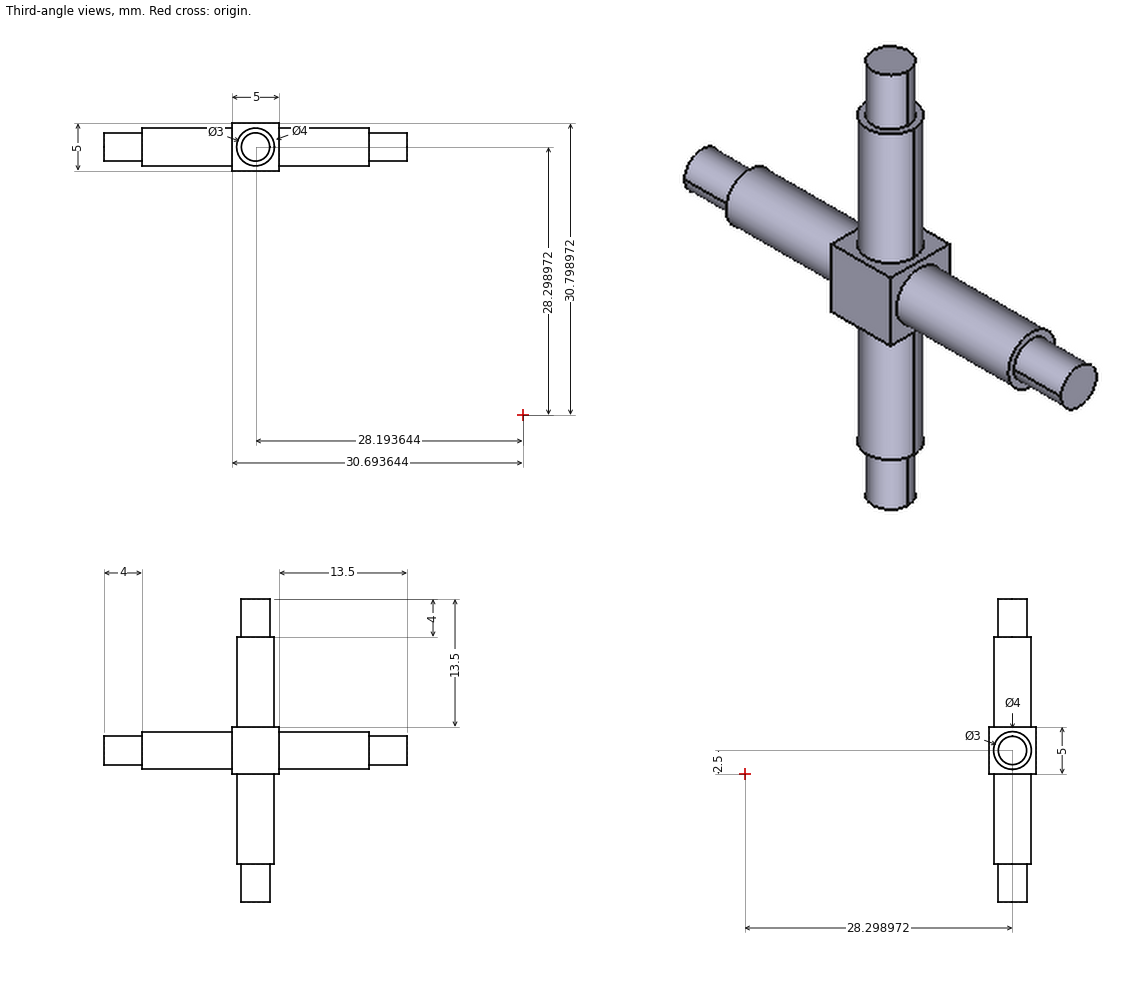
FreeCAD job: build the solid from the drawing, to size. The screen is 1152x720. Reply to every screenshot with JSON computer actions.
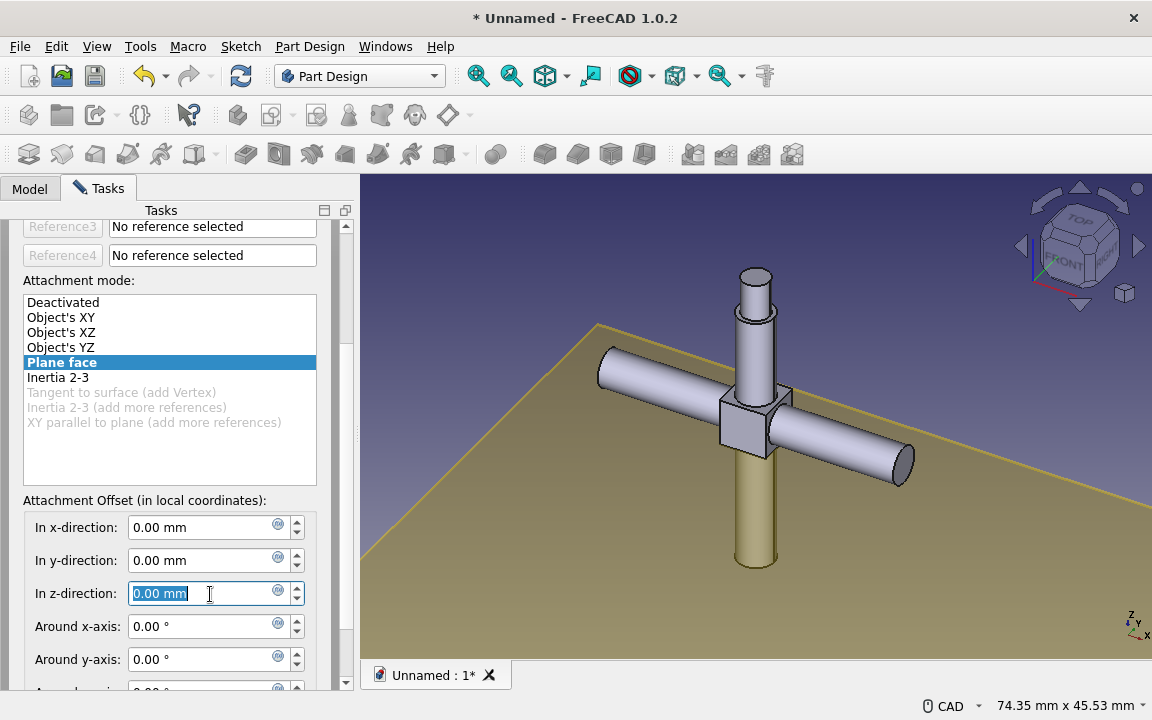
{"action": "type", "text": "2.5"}
{"action": "key", "text": "Tab"}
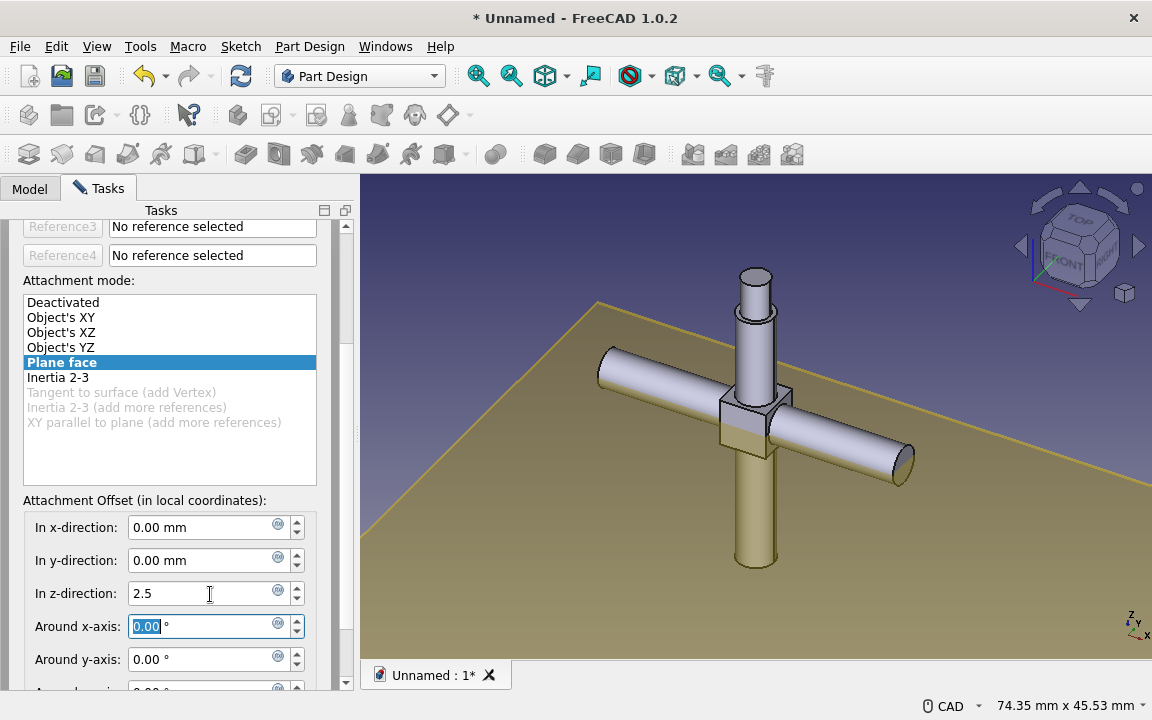
{"action": "scroll", "coordinate": [346, 455], "scroll_direction": "up", "scroll_amount": 4}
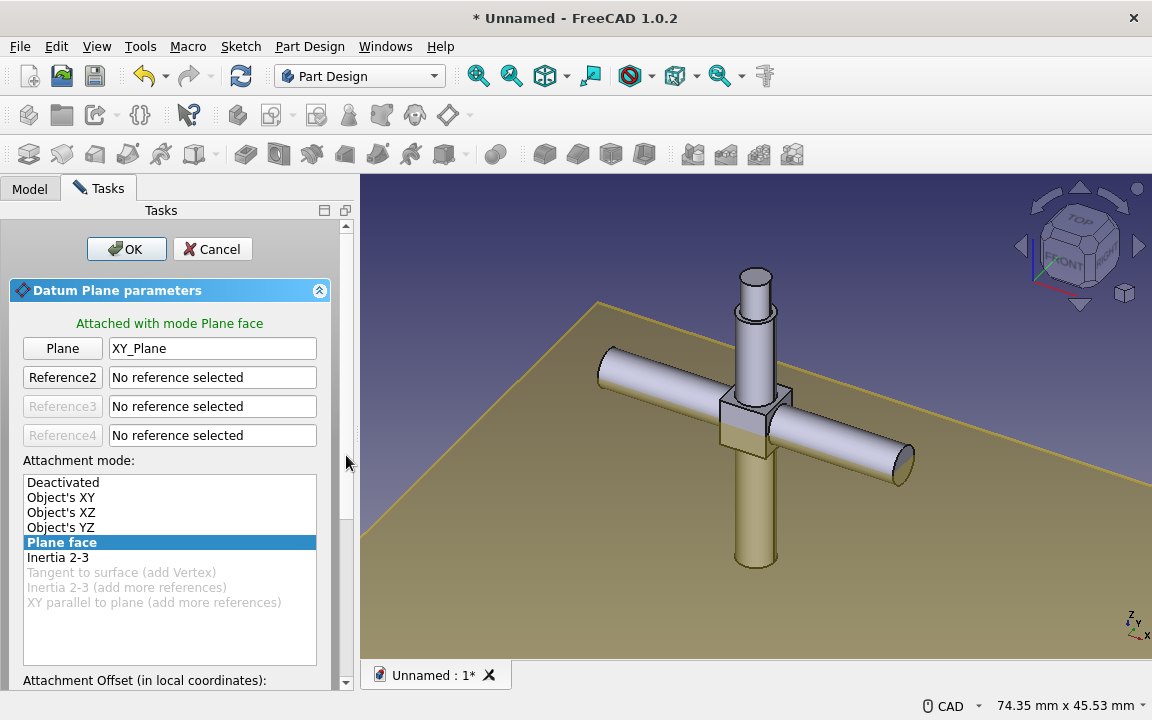
{"action": "left_click", "coordinate": [127, 249]}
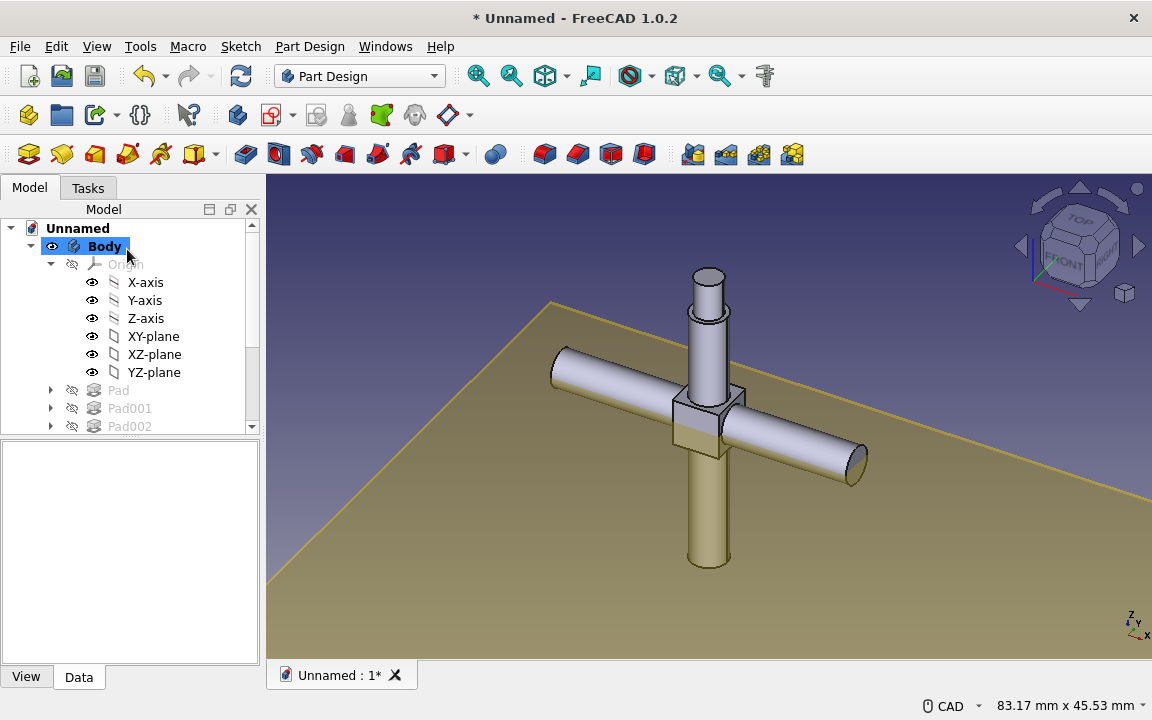
{"action": "scroll", "coordinate": [101, 332], "scroll_direction": "down", "scroll_amount": 3}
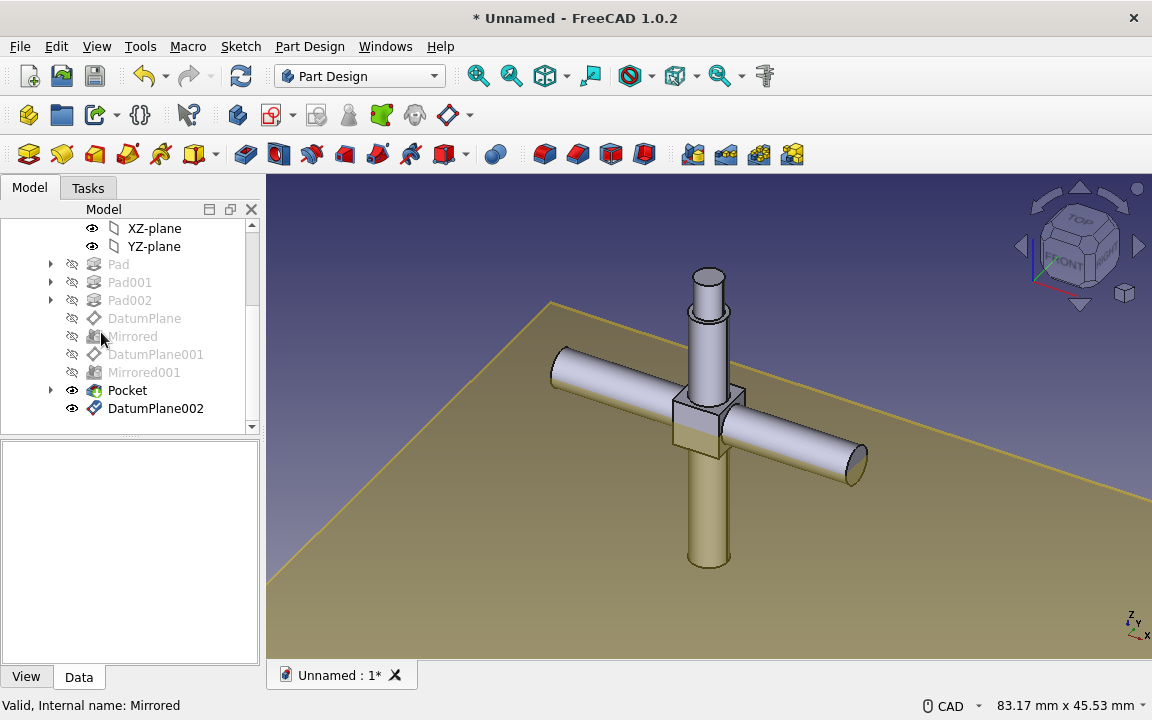
{"action": "left_click", "coordinate": [117, 390]}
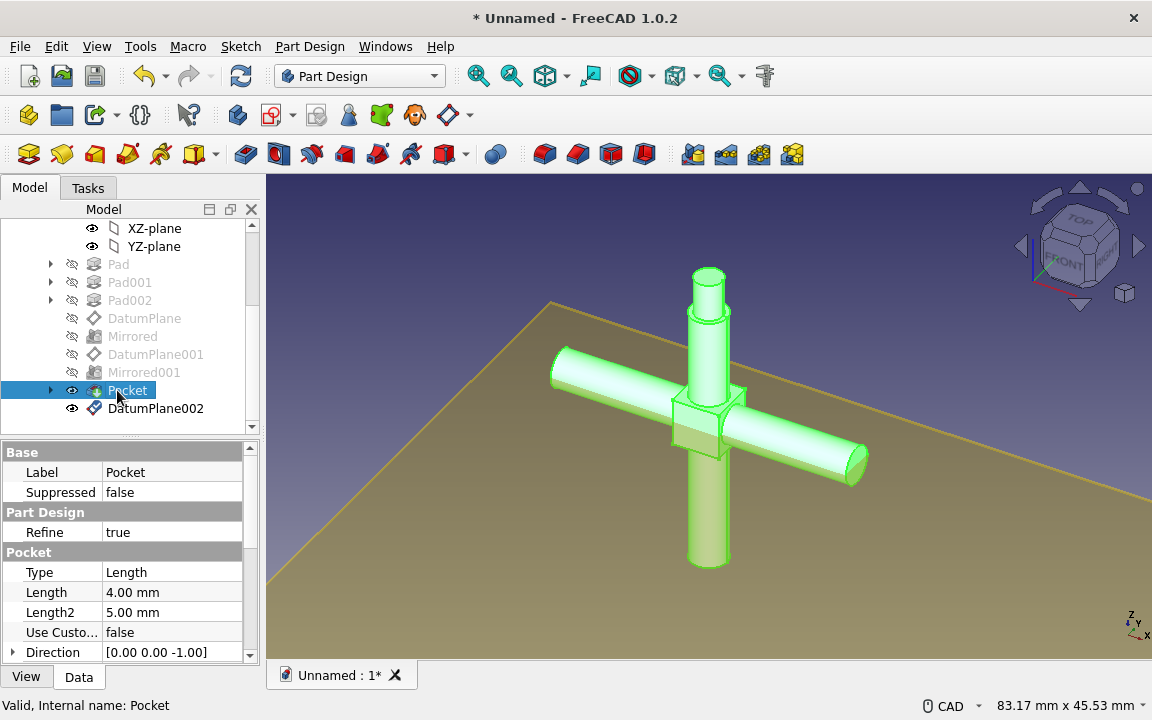
{"action": "left_click", "coordinate": [693, 154]}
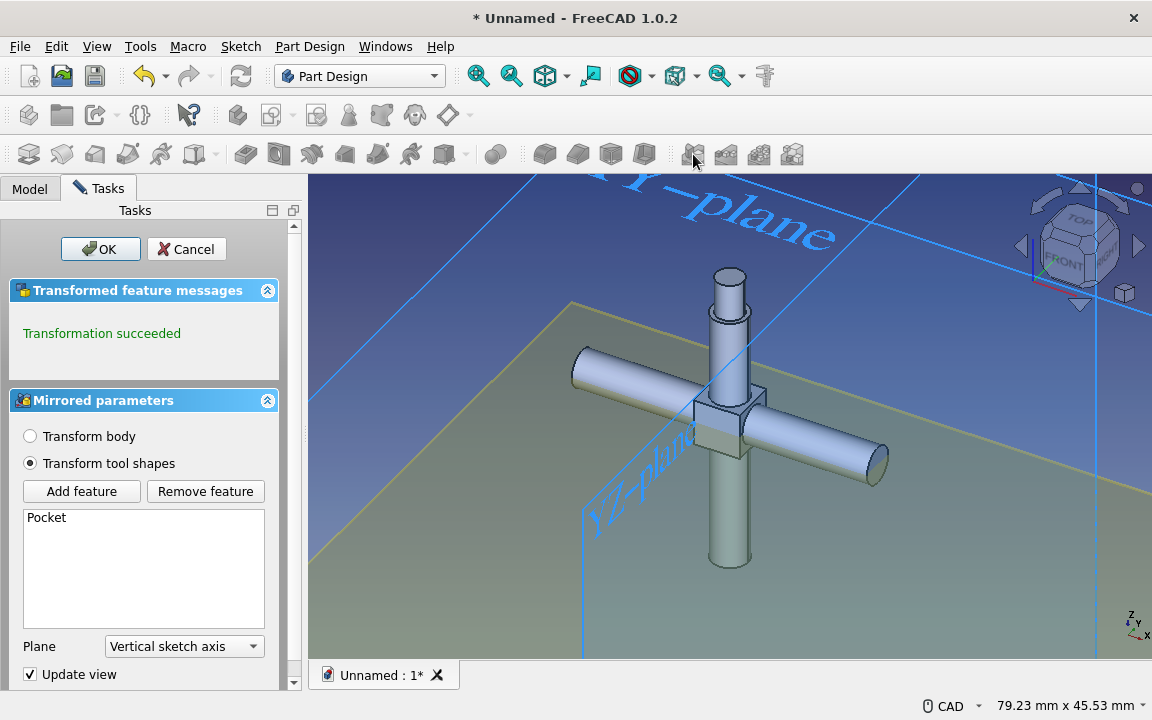
{"action": "left_click", "coordinate": [185, 646]}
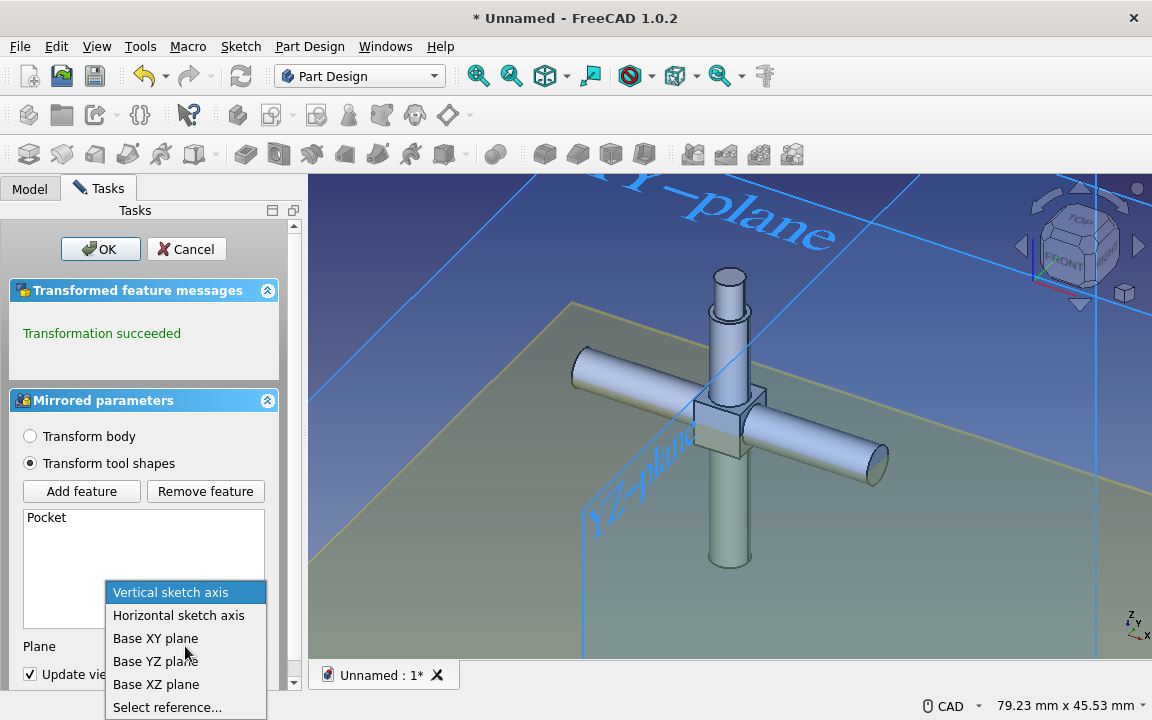
{"action": "left_click", "coordinate": [184, 708]}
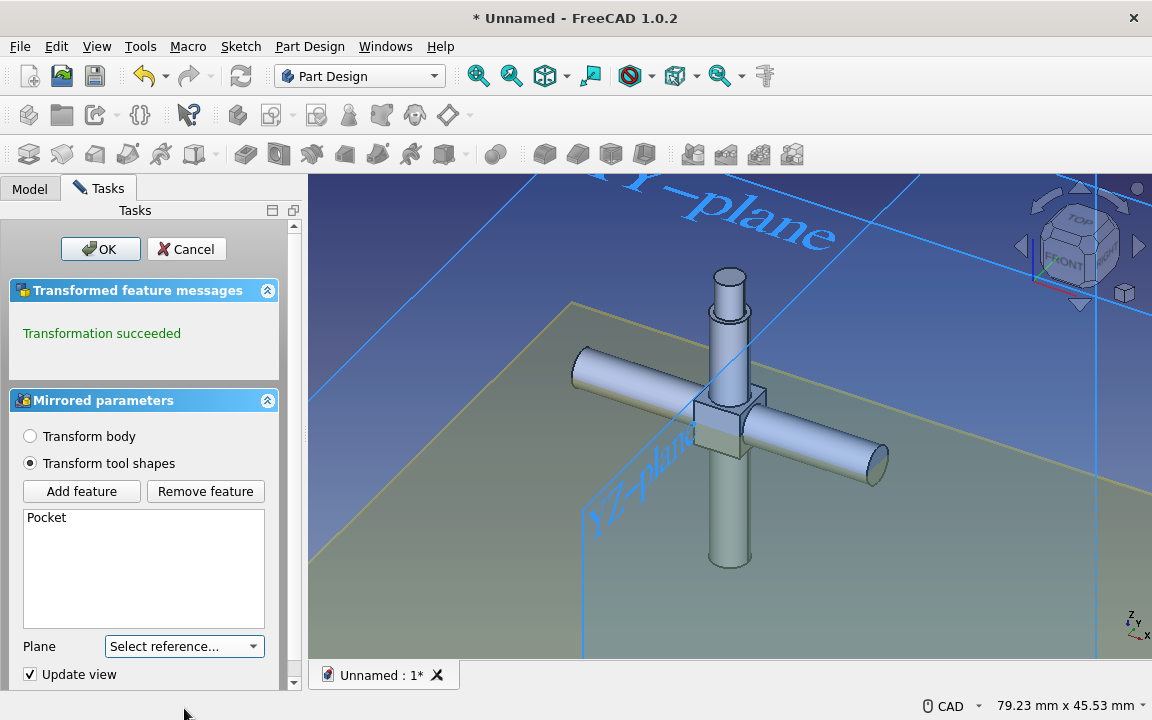
{"action": "left_click", "coordinate": [30, 188]}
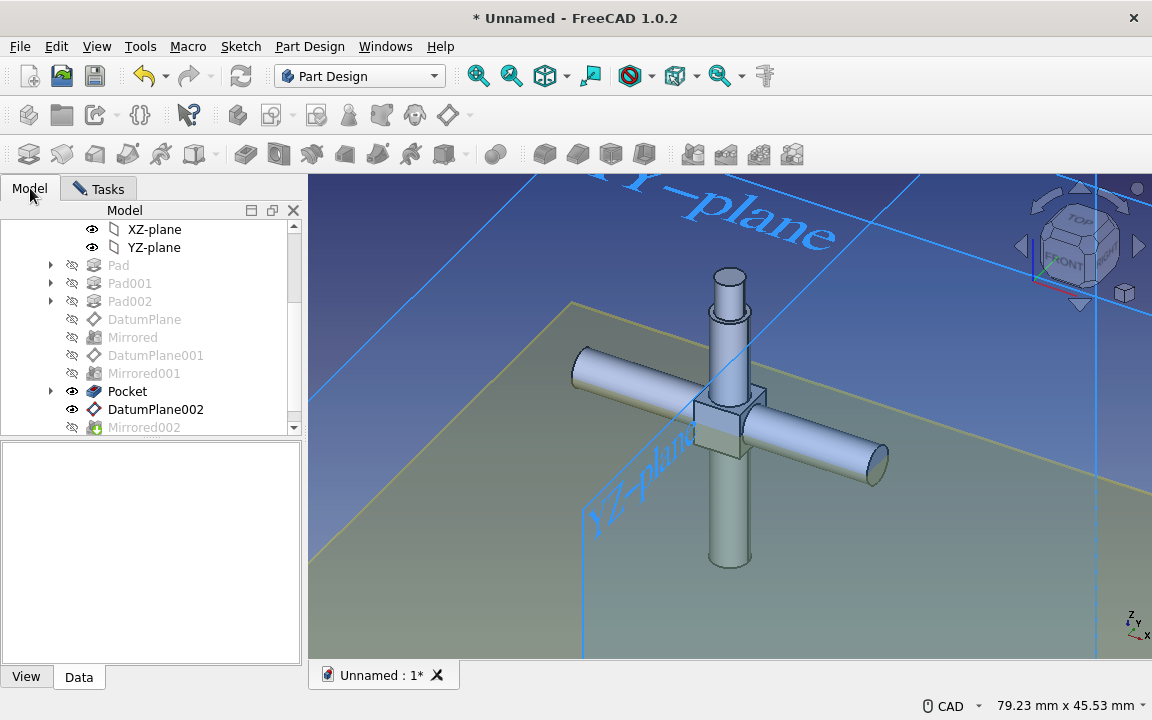
{"action": "left_click", "coordinate": [117, 409]}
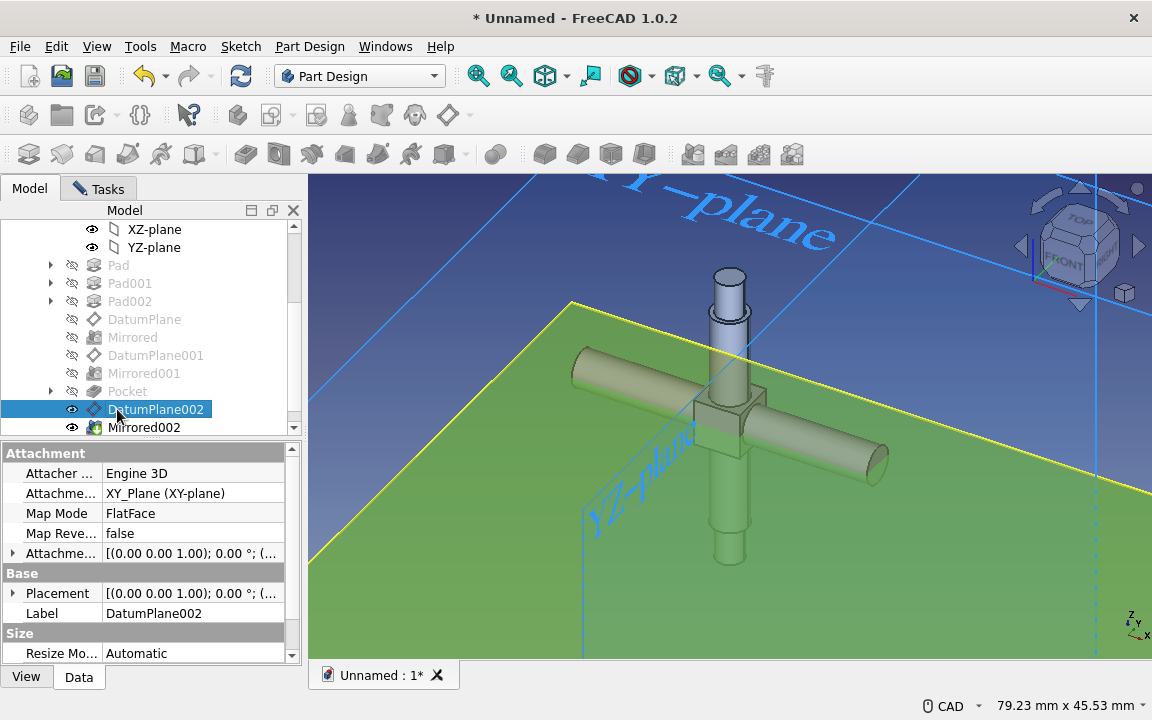
{"action": "left_click", "coordinate": [98, 188]}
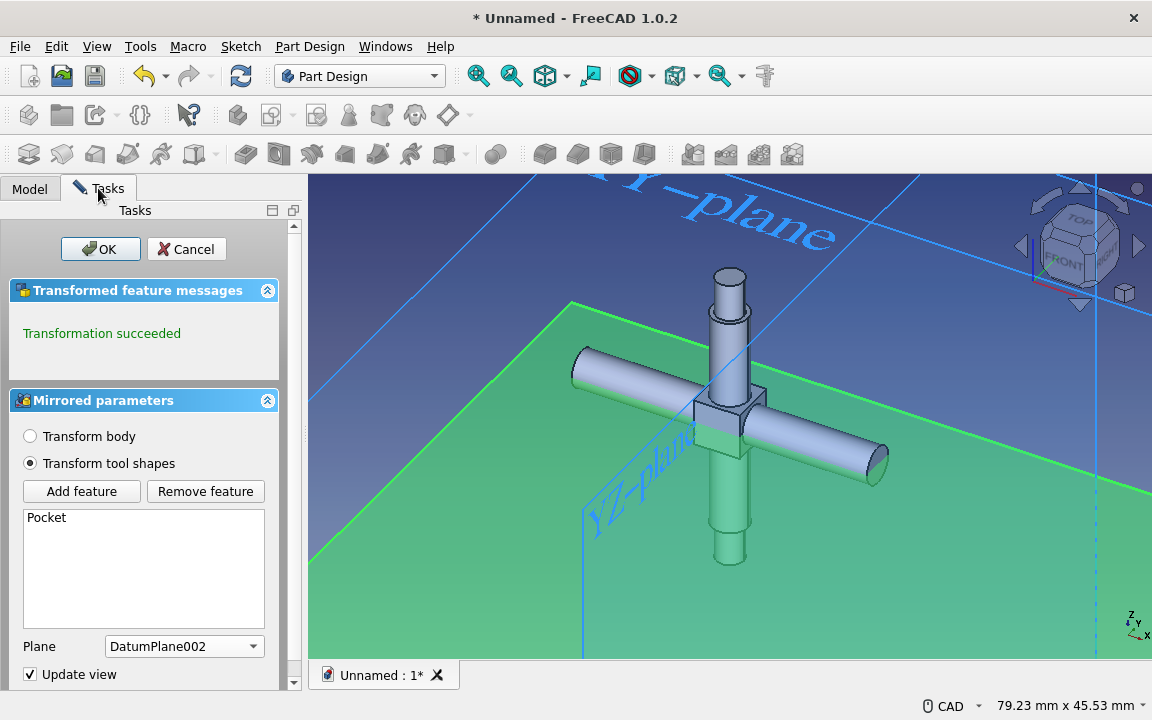
{"action": "left_click", "coordinate": [101, 249]}